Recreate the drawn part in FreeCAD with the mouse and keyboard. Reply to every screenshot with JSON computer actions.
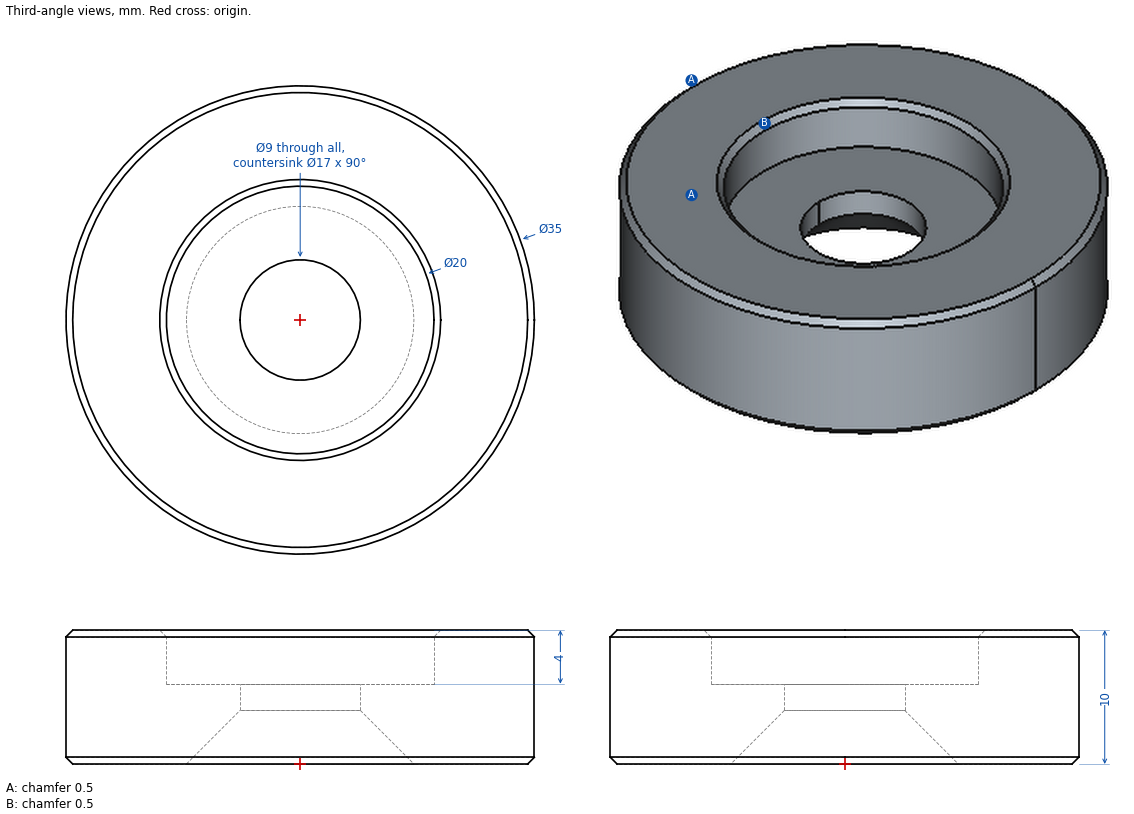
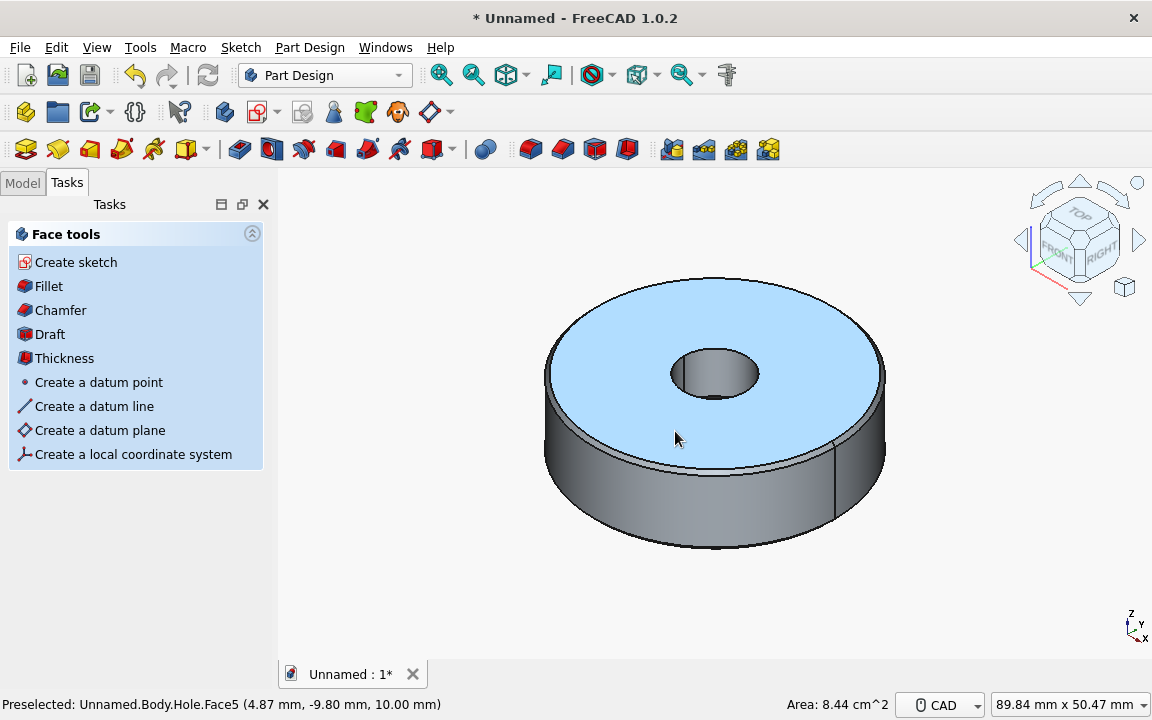
{"action": "left_click", "coordinate": [258, 112]}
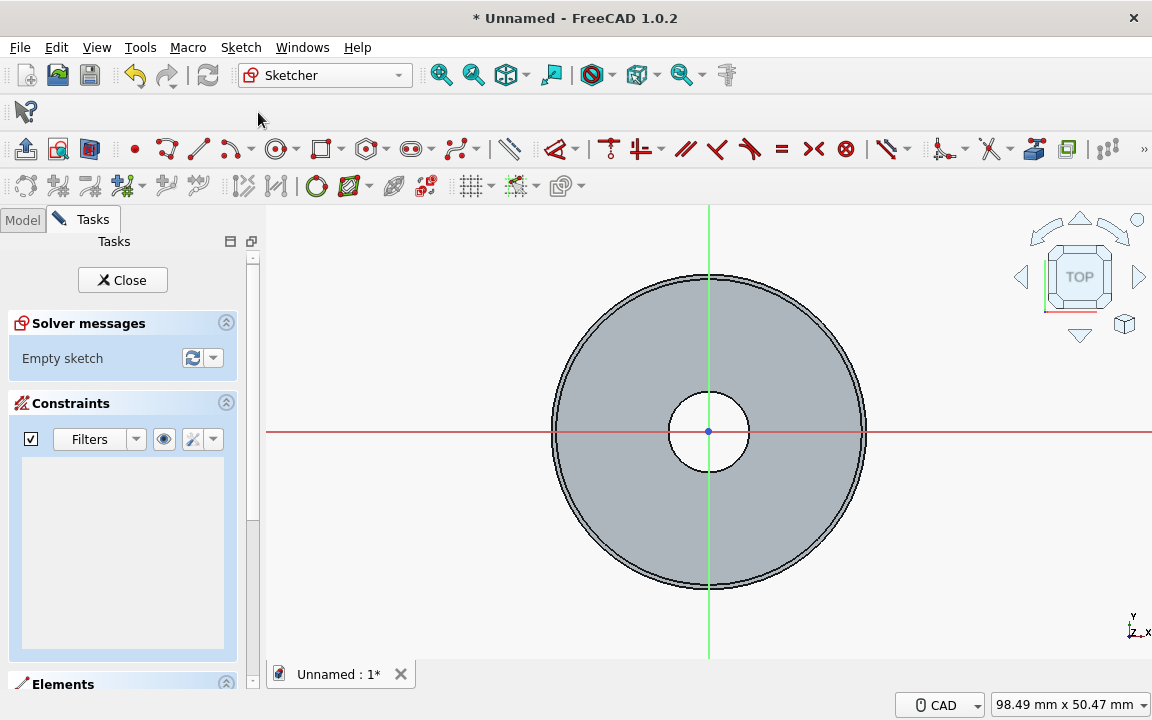
{"action": "scroll", "coordinate": [848, 432], "scroll_direction": "up", "scroll_amount": 2}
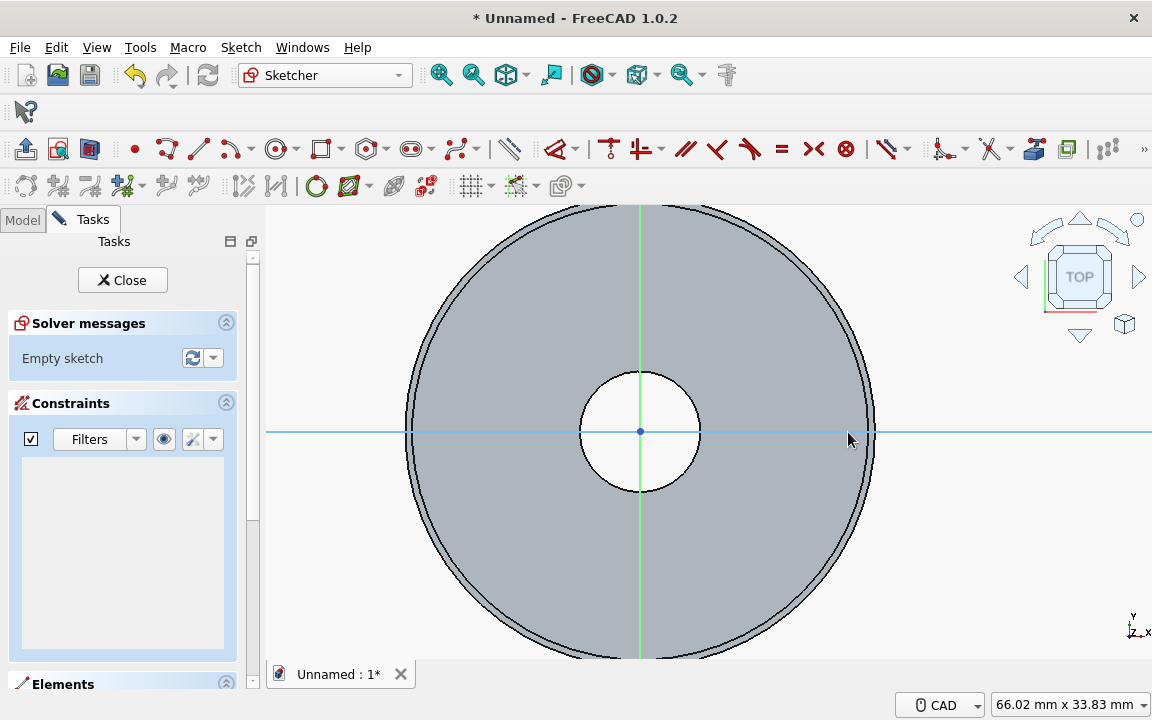
{"action": "left_click", "coordinate": [276, 150]}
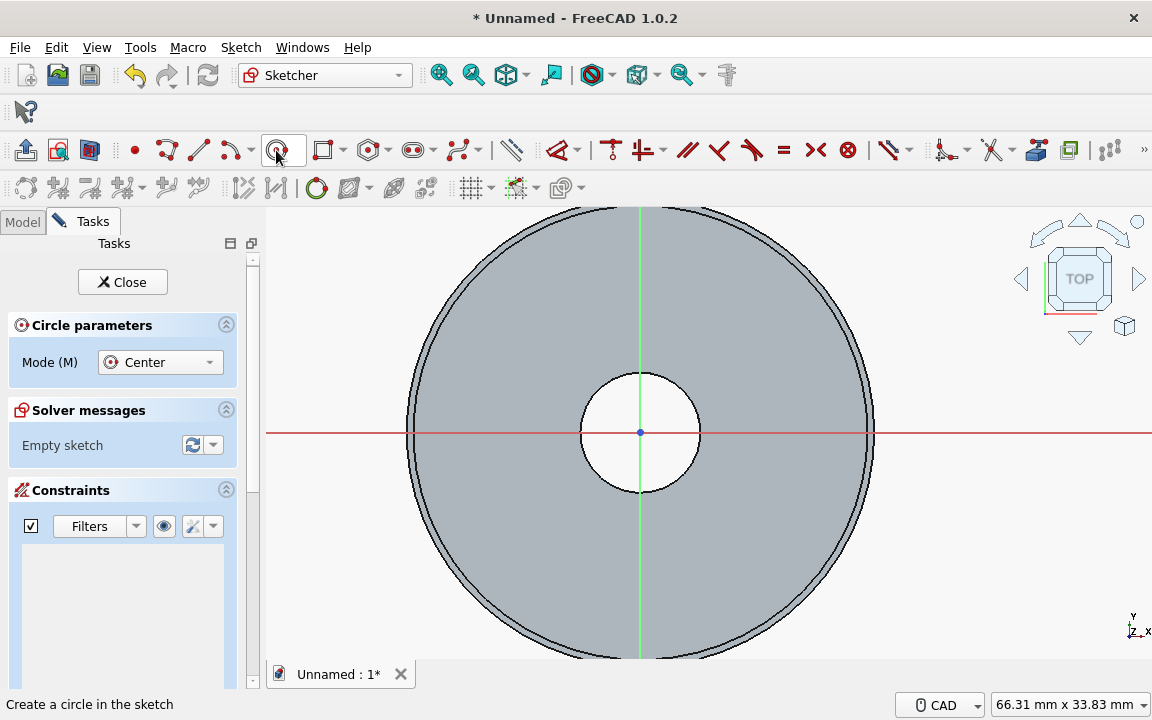
{"action": "left_click", "coordinate": [640, 433]}
{"action": "mouse_move", "coordinate": [735, 338]}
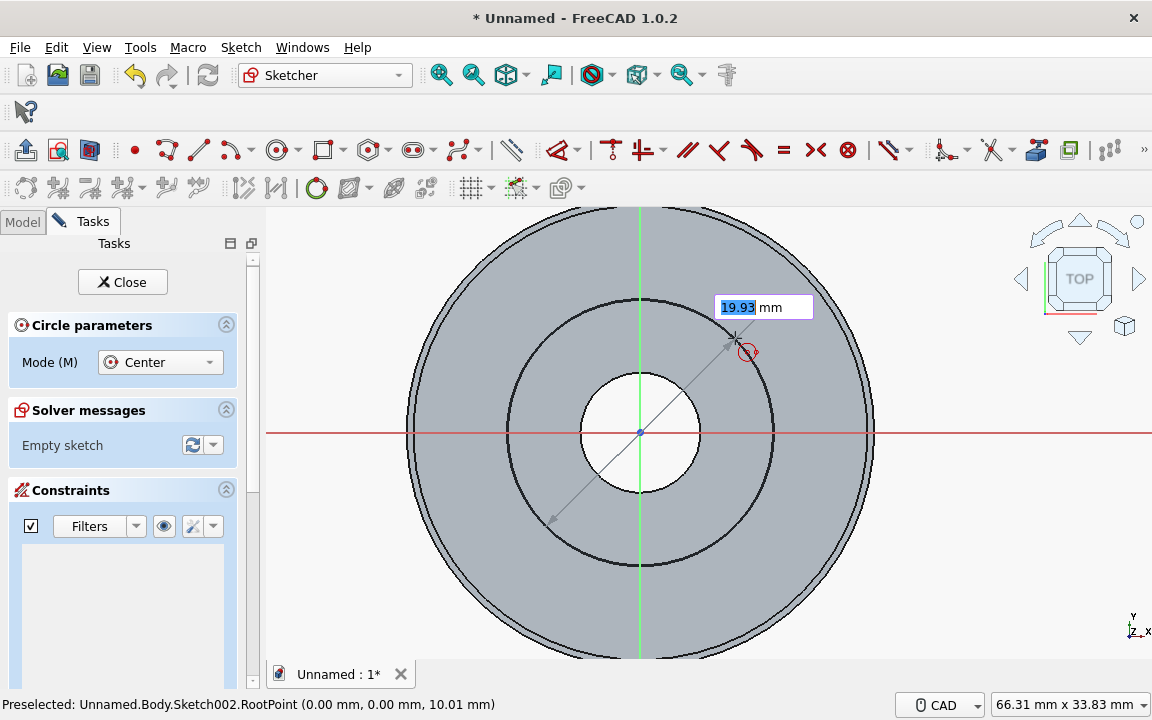
{"action": "type", "text": "20"}
{"action": "key", "text": "Return"}
{"action": "key", "text": "Escape"}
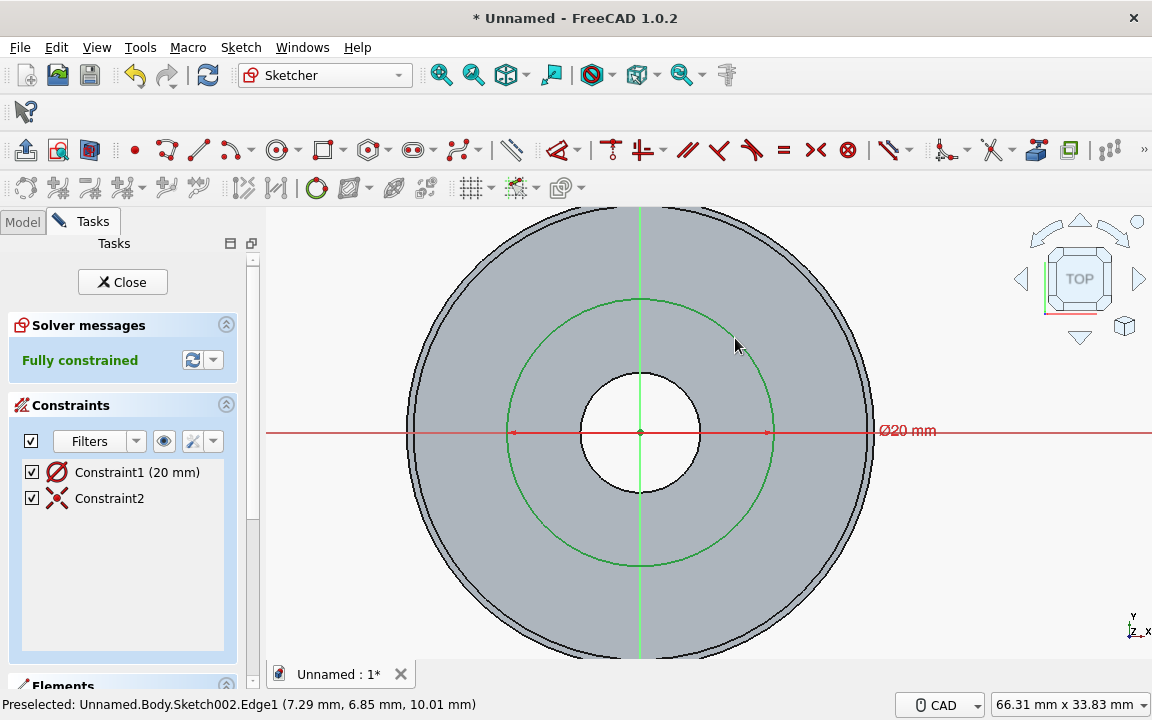
{"action": "left_click", "coordinate": [123, 282]}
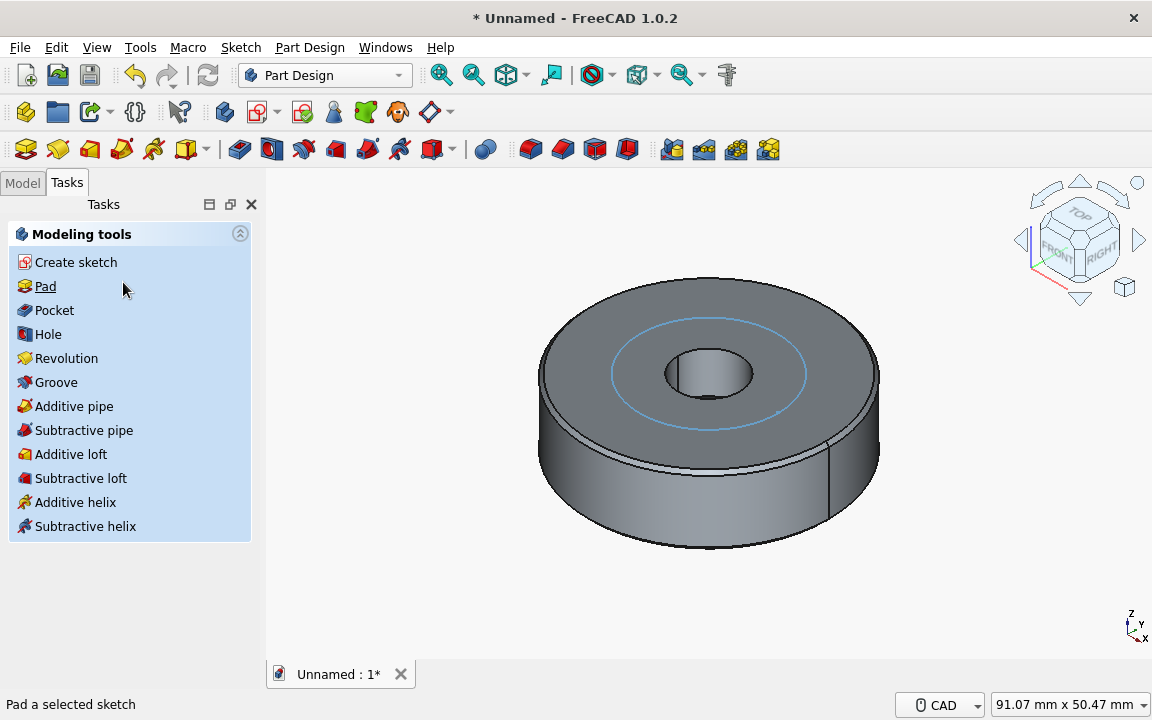
{"action": "left_click", "coordinate": [240, 150]}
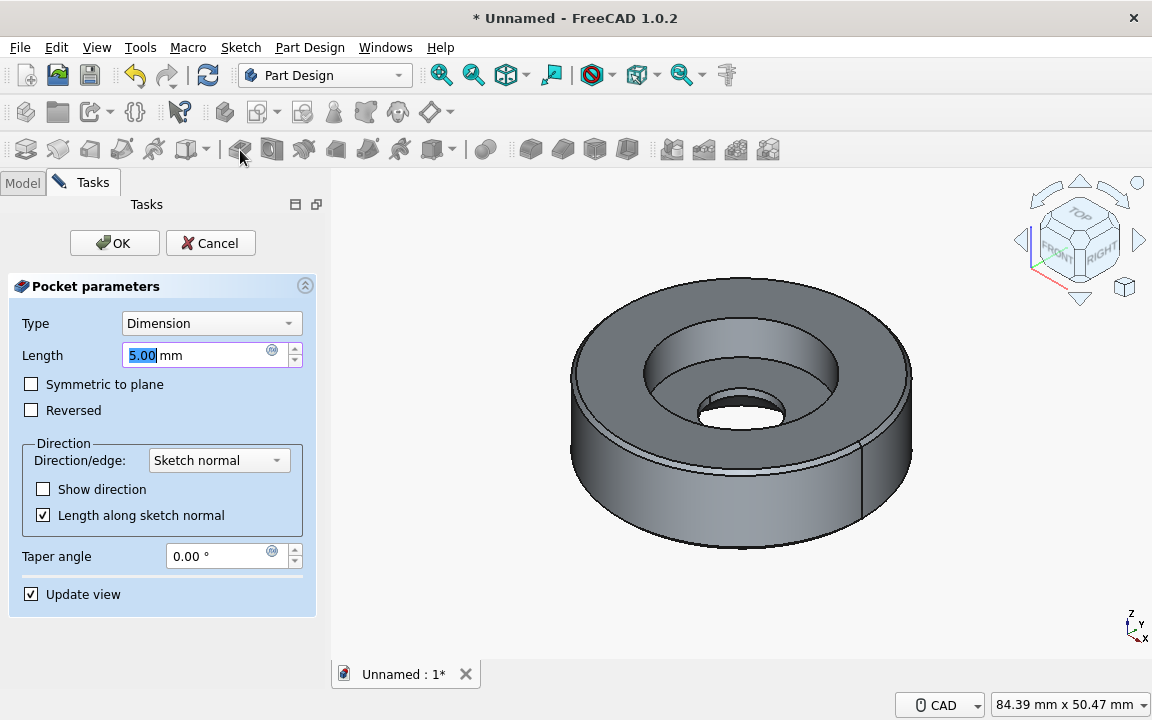
{"action": "type", "text": "4"}
{"action": "key", "text": "Tab"}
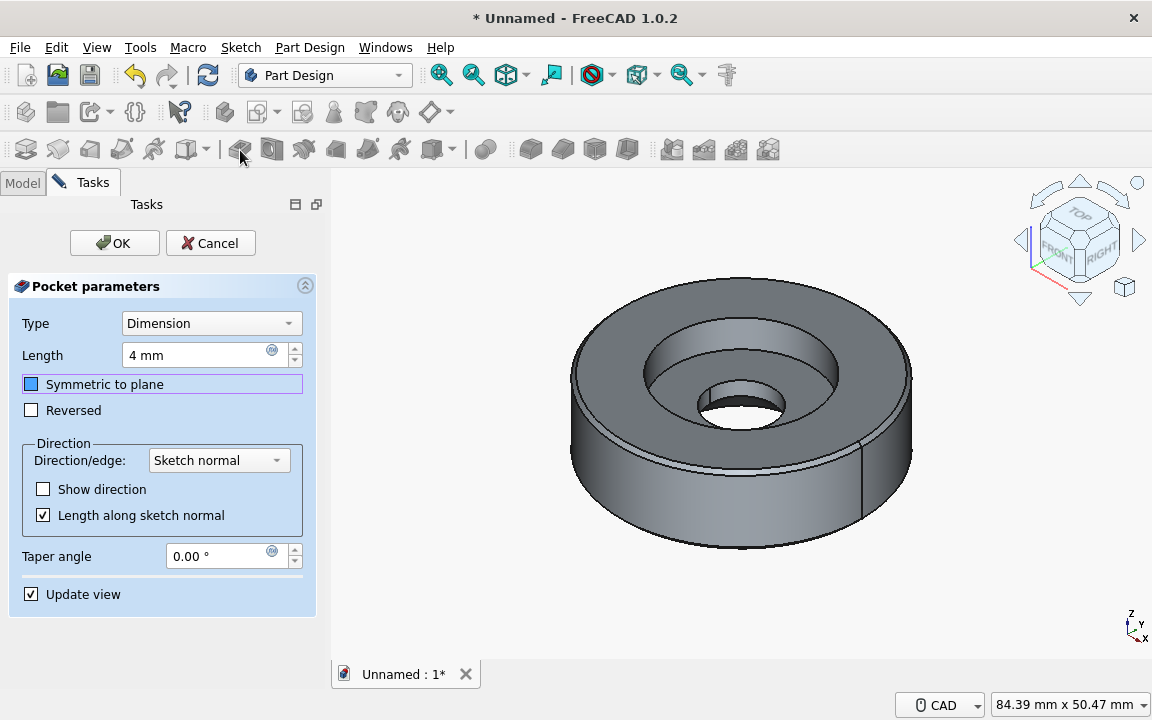
{"action": "left_click", "coordinate": [115, 243]}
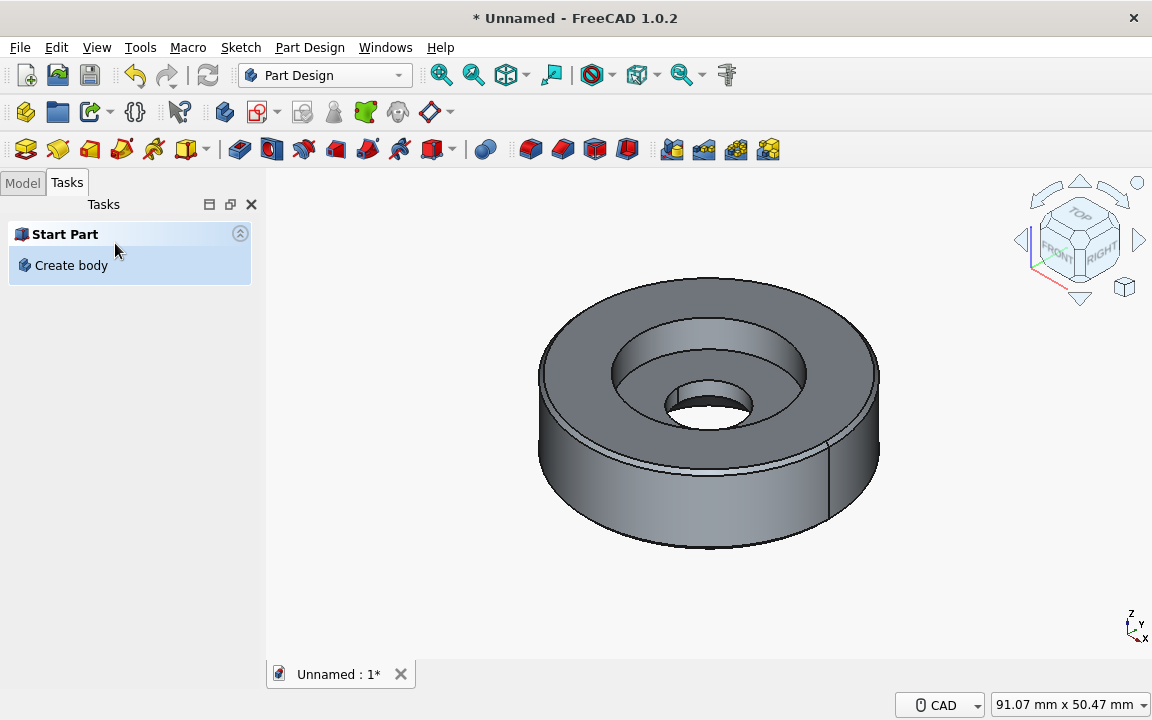
{"action": "left_click", "coordinate": [640, 333]}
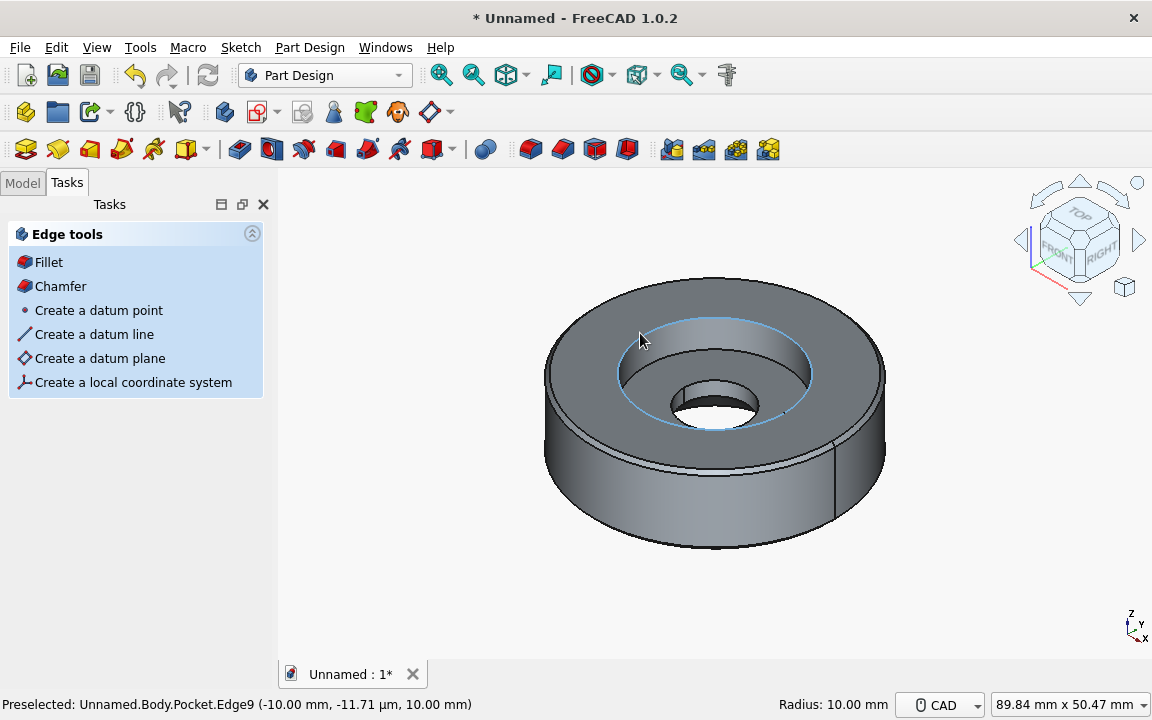
{"action": "left_click", "coordinate": [564, 150]}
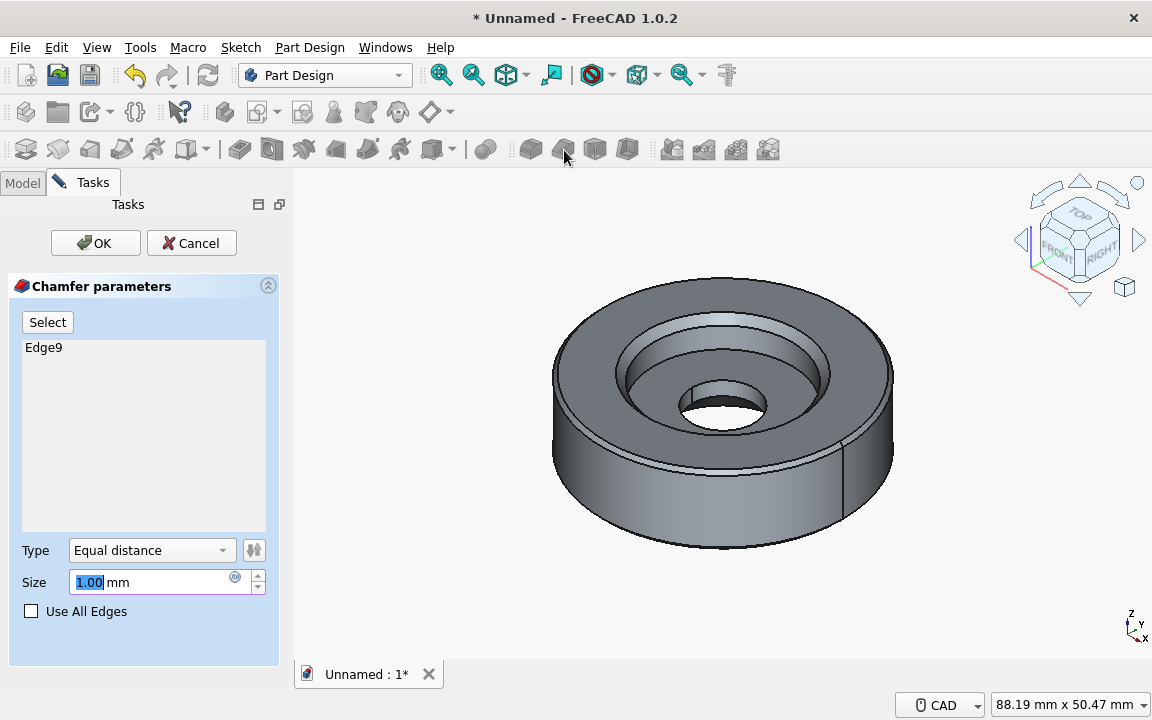
{"action": "type", "text": "0.5"}
{"action": "key", "text": "Tab"}